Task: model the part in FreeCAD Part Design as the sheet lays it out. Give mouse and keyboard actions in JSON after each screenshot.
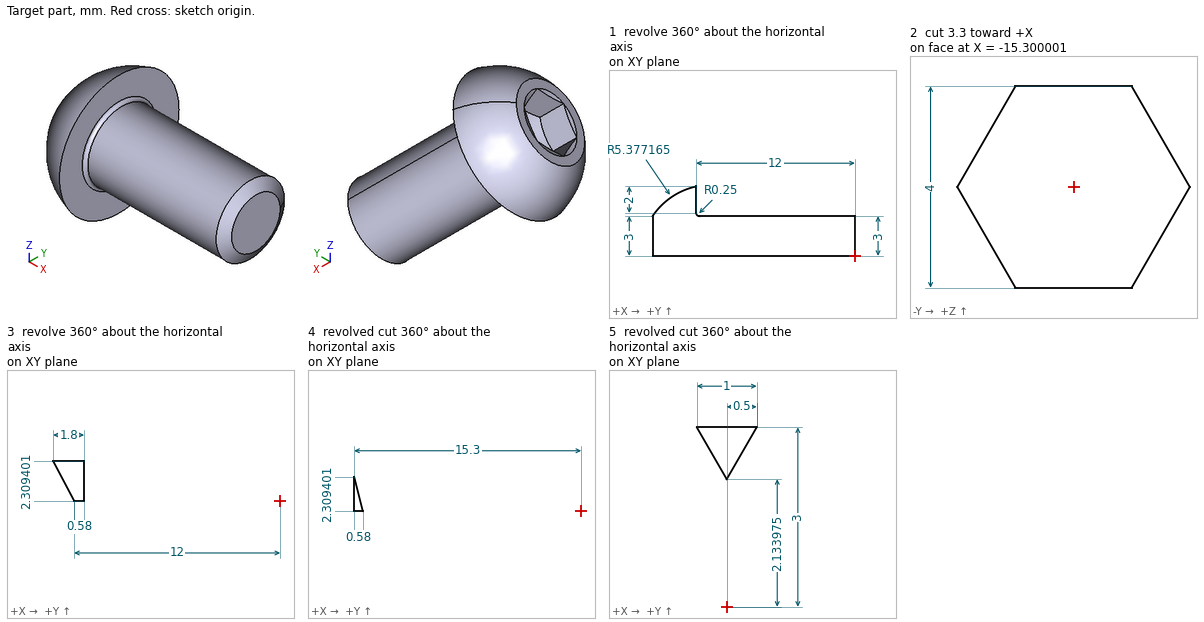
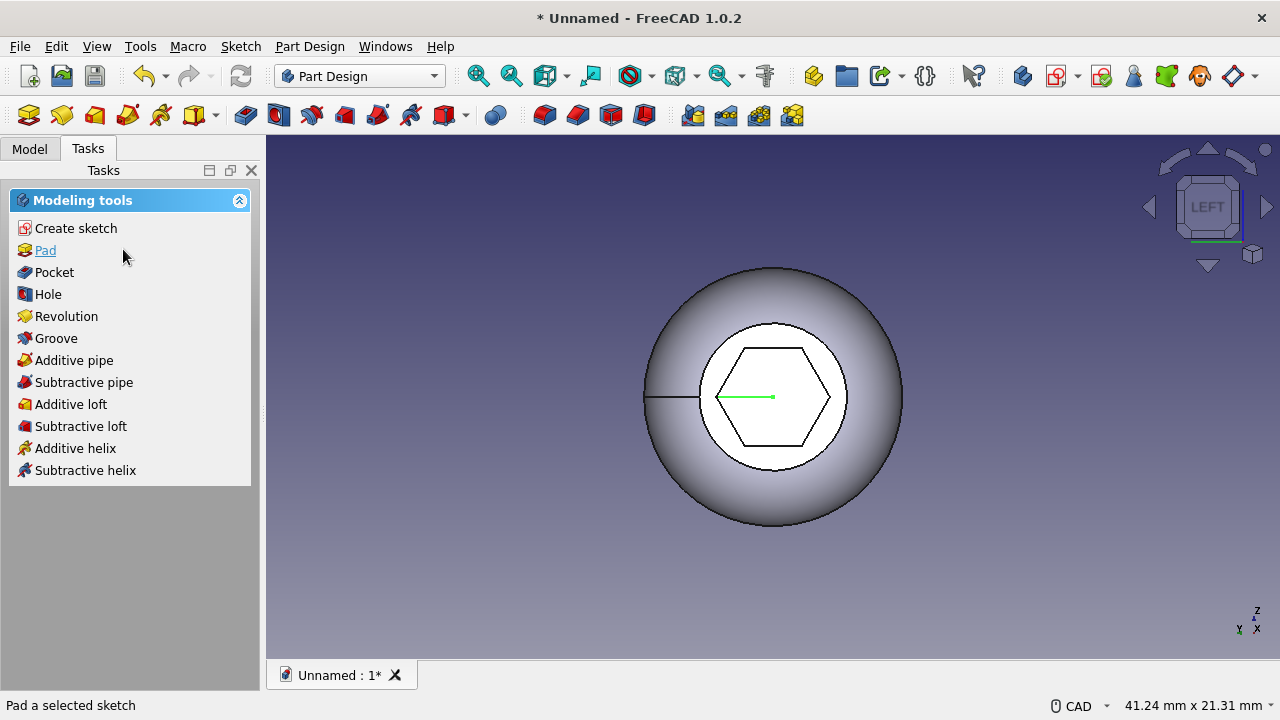
{"action": "left_click", "coordinate": [62, 116]}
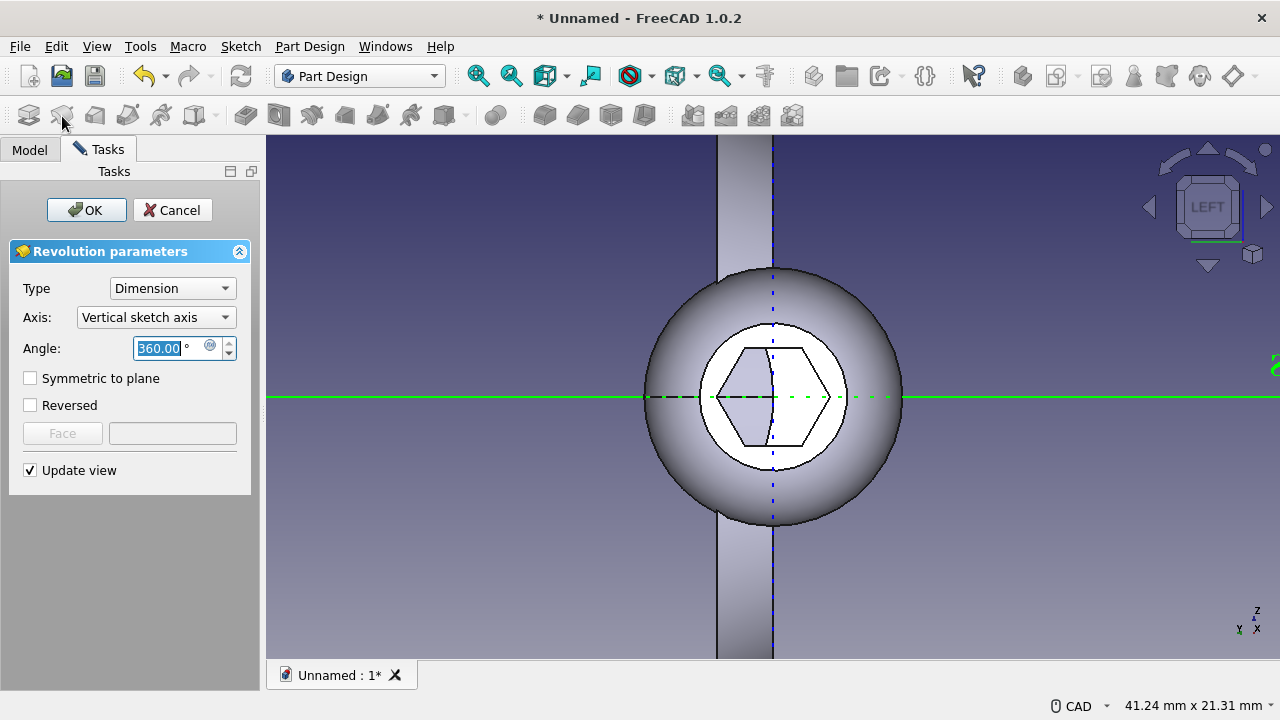
{"action": "left_click", "coordinate": [157, 318]}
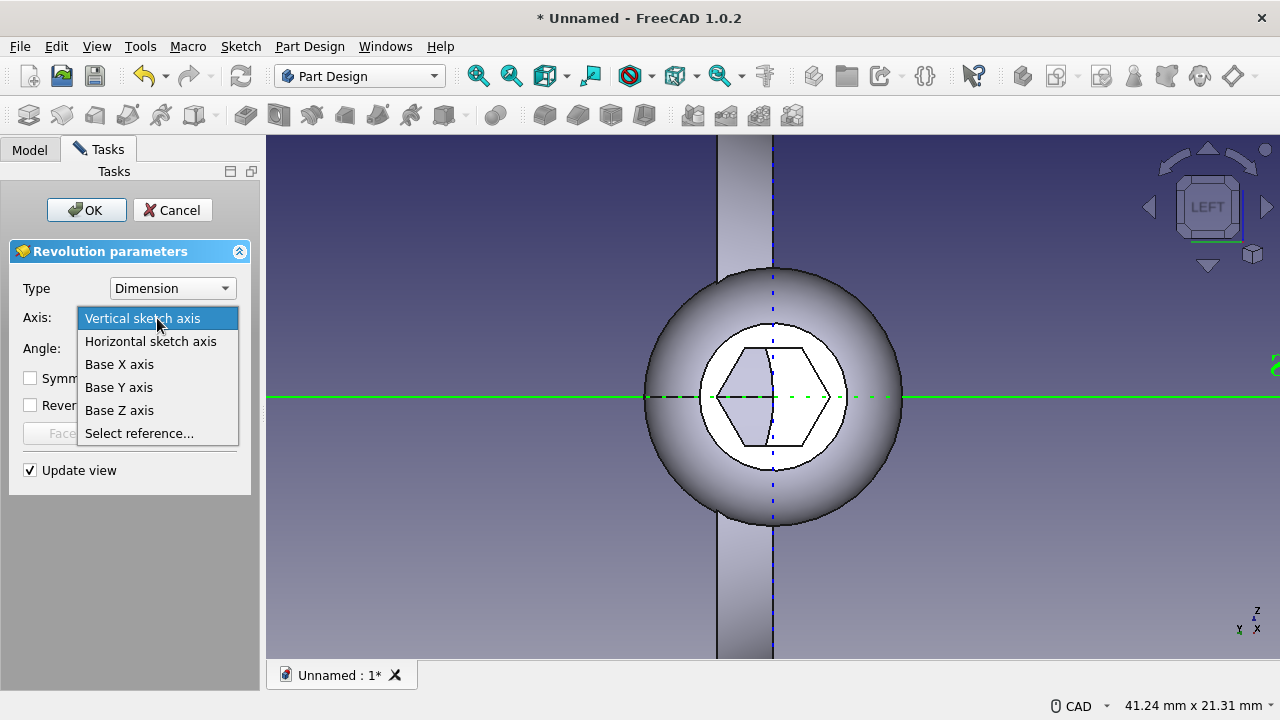
{"action": "left_click", "coordinate": [156, 342]}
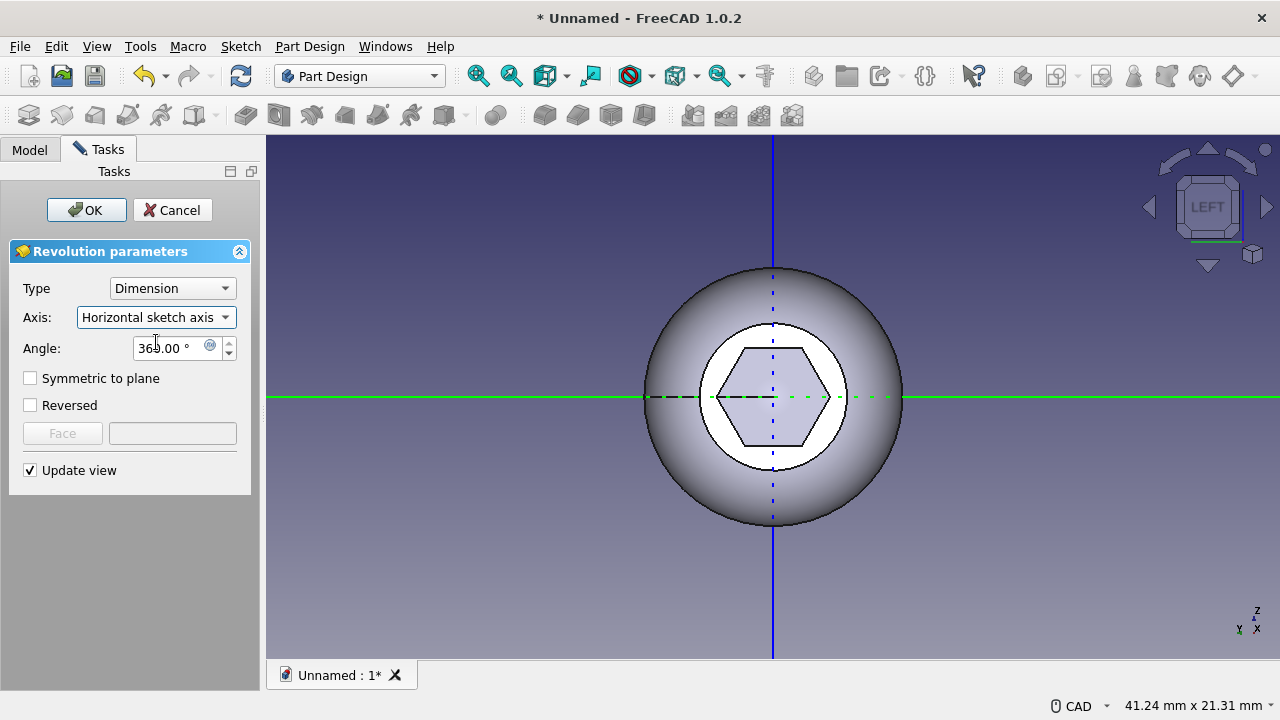
{"action": "left_click", "coordinate": [87, 210]}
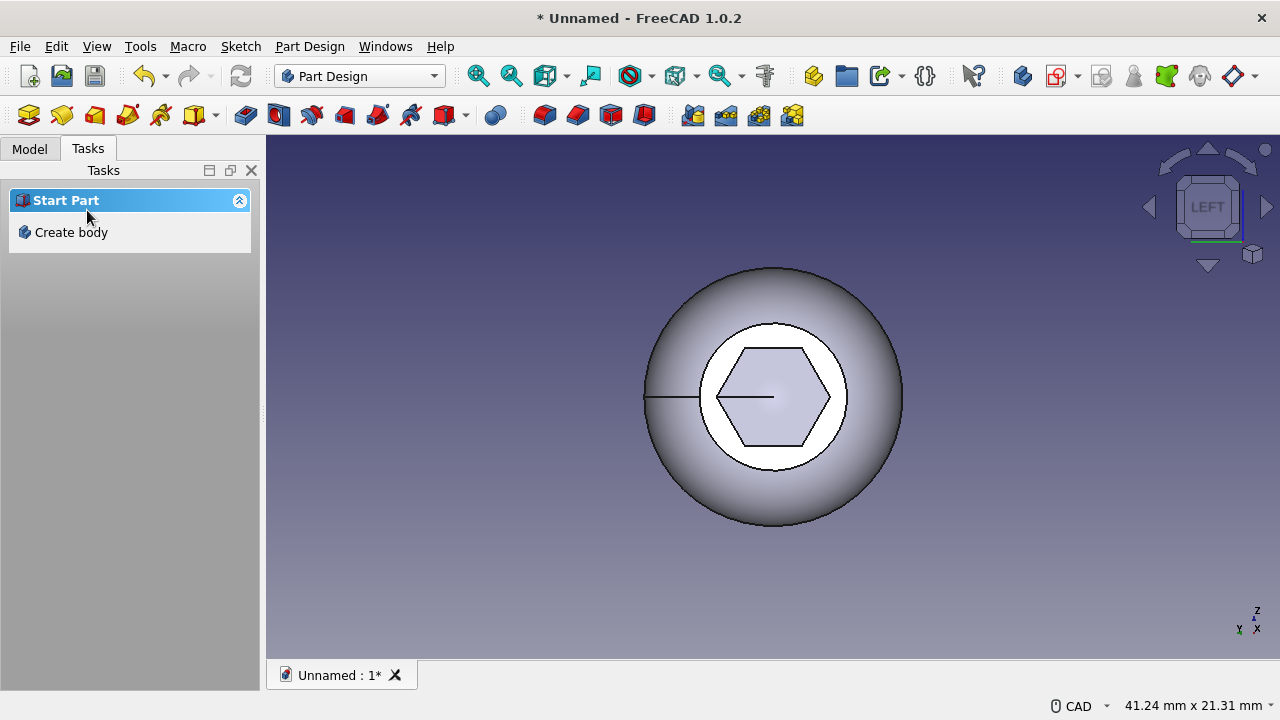
{"action": "left_click", "coordinate": [1056, 76]}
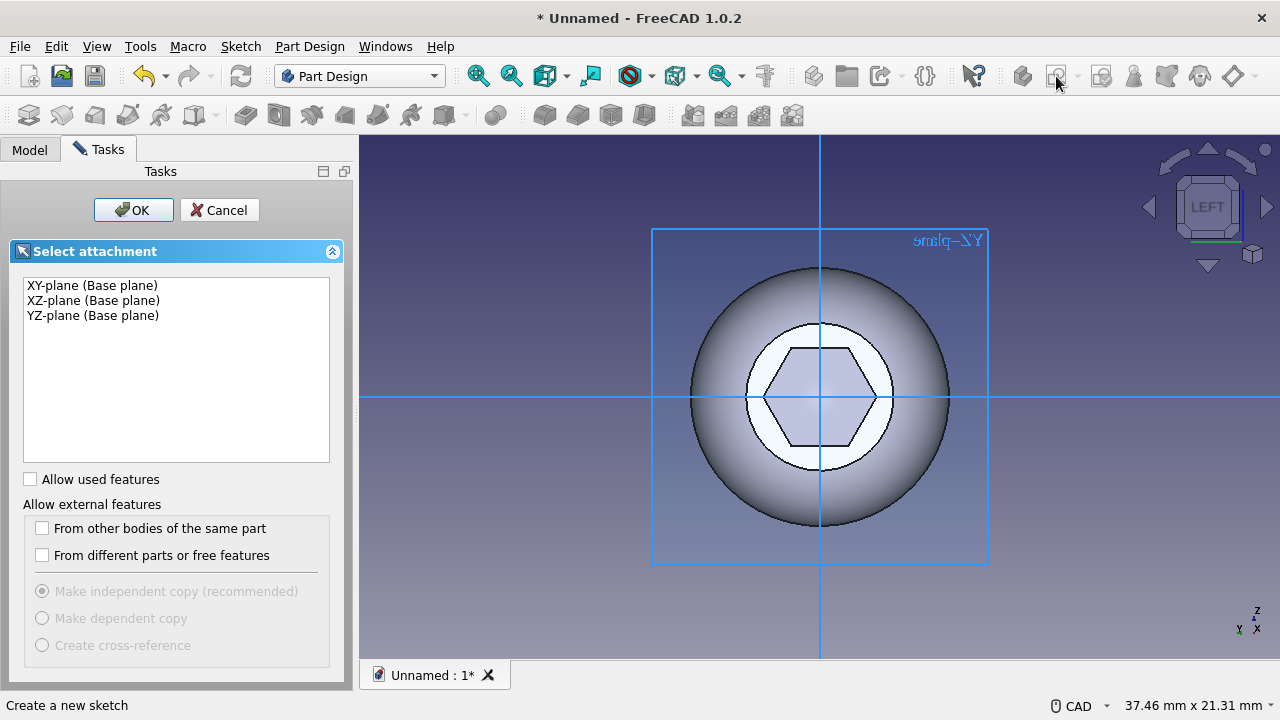
{"action": "left_click", "coordinate": [84, 286]}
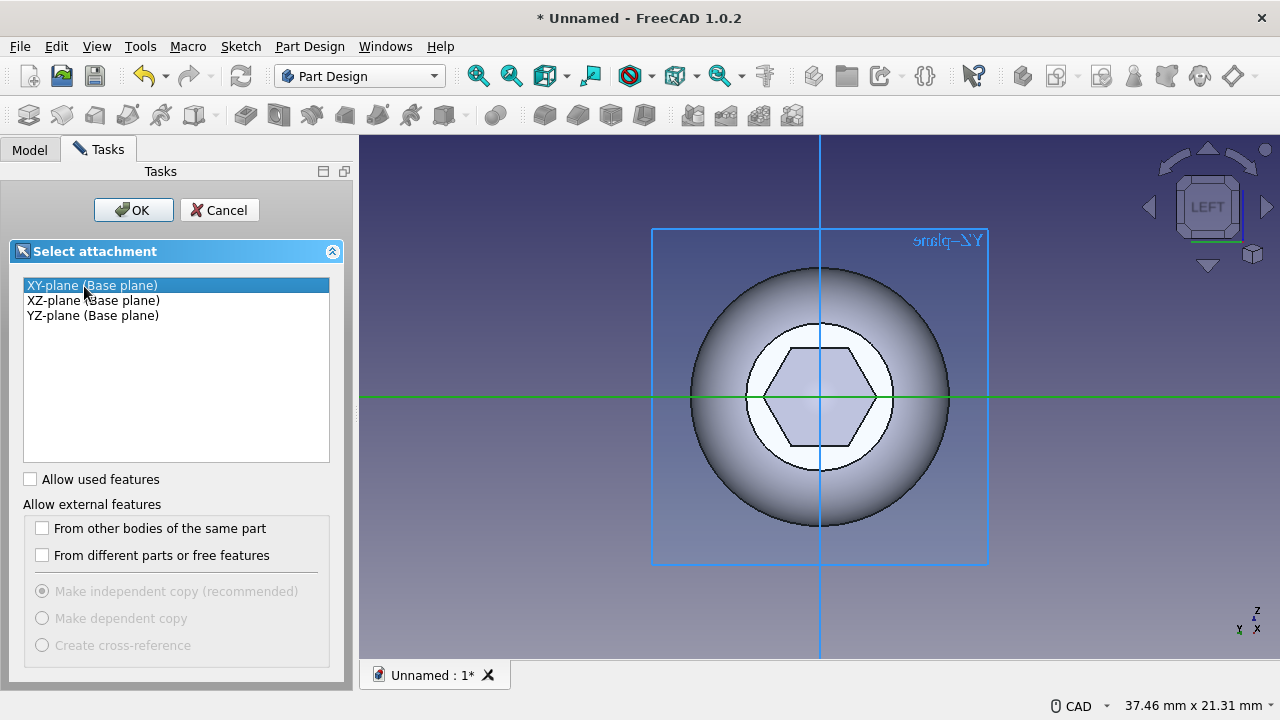
{"action": "left_click", "coordinate": [134, 210]}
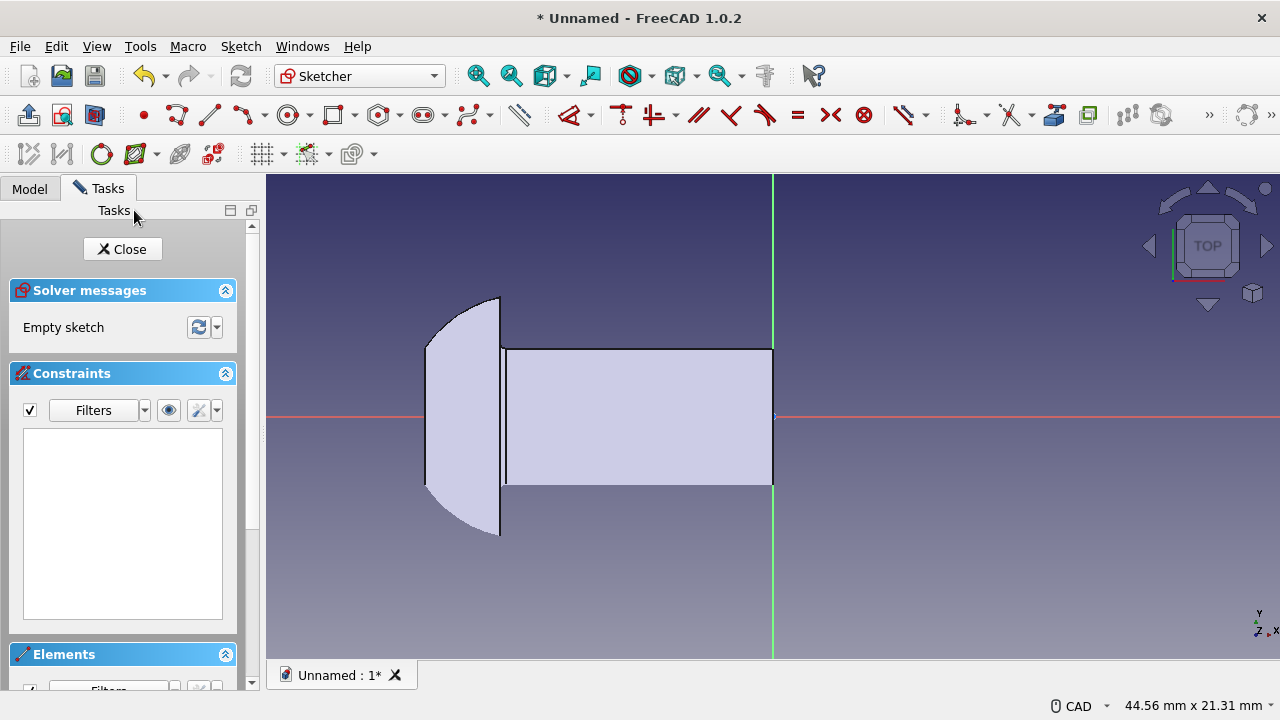
{"action": "left_click", "coordinate": [95, 116]}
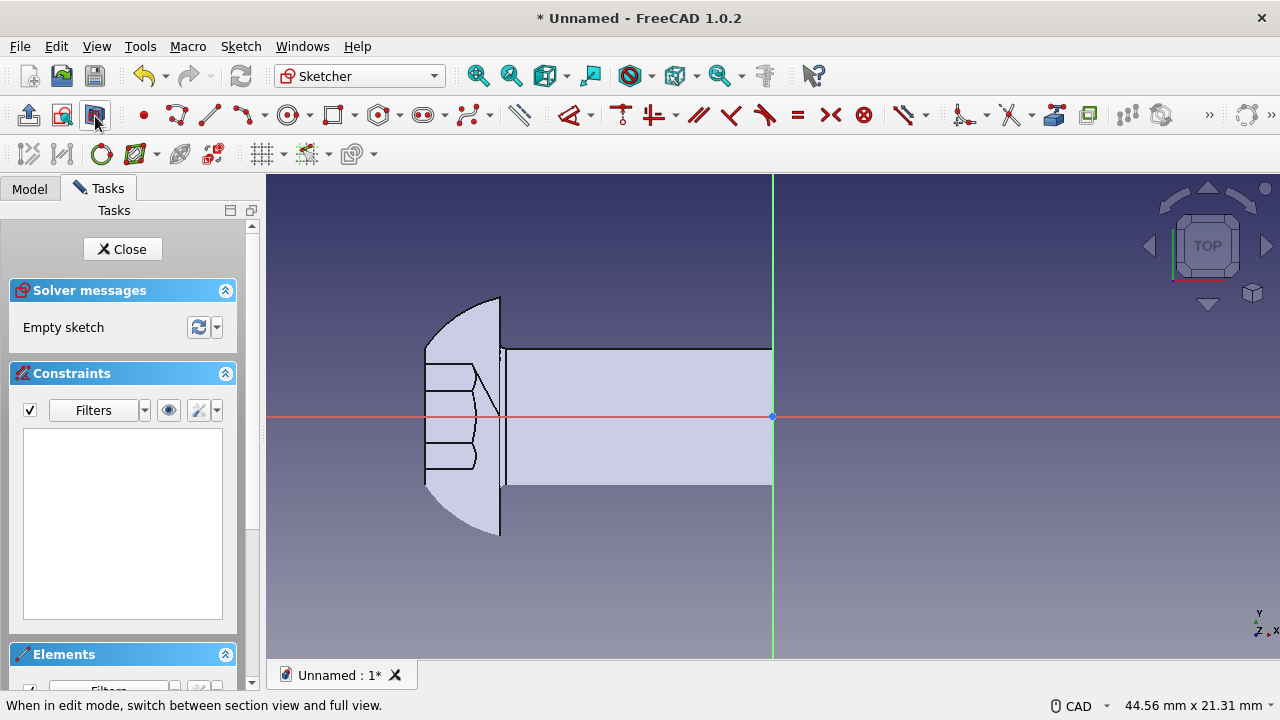
{"action": "scroll", "coordinate": [377, 385], "scroll_direction": "up", "scroll_amount": 9}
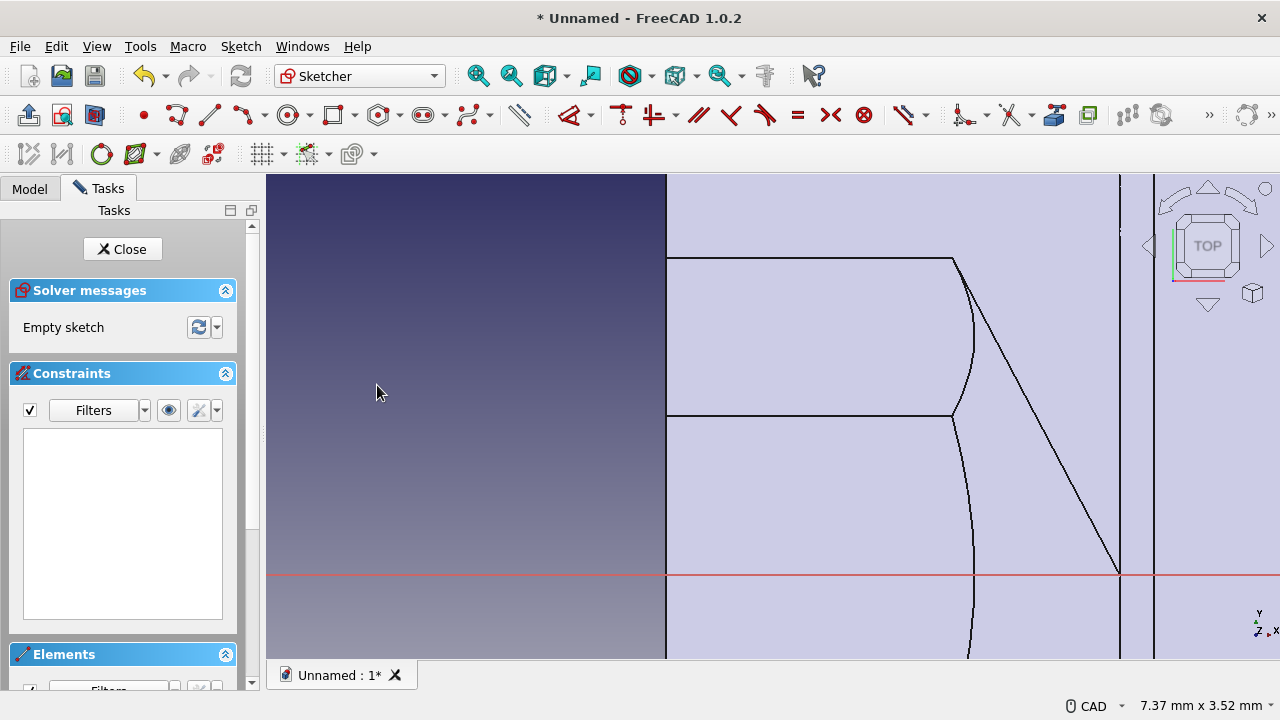
{"action": "left_click", "coordinate": [177, 116]}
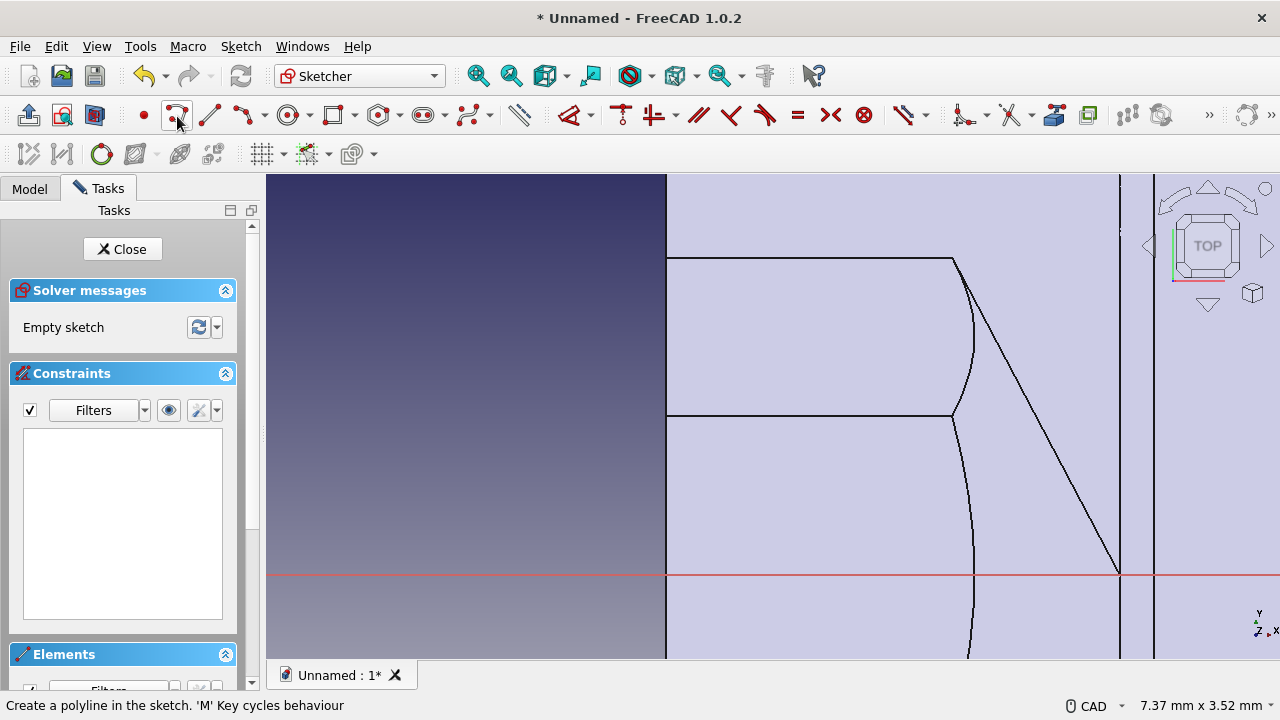
{"action": "left_click", "coordinate": [746, 575]}
{"action": "left_click", "coordinate": [666, 258]}
{"action": "left_click", "coordinate": [666, 566]}
{"action": "left_click", "coordinate": [746, 575]}
{"action": "key", "text": "Escape"}
{"action": "key", "text": "Escape"}